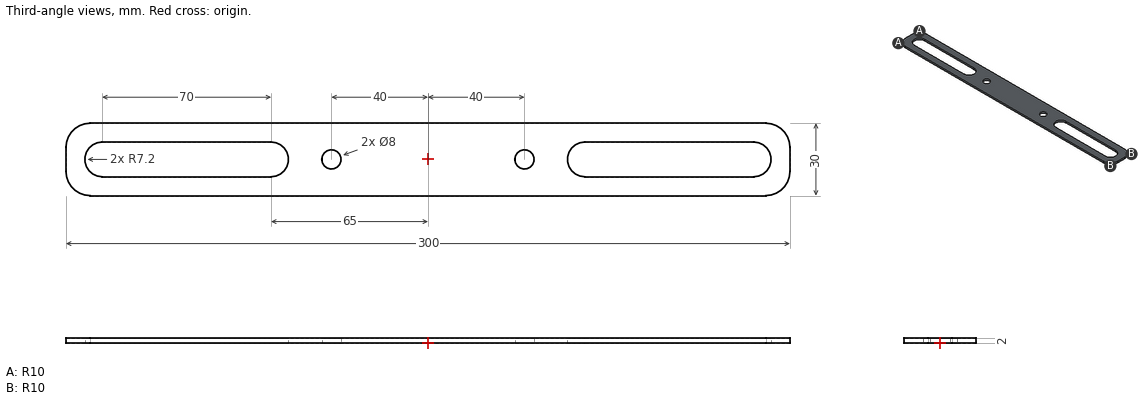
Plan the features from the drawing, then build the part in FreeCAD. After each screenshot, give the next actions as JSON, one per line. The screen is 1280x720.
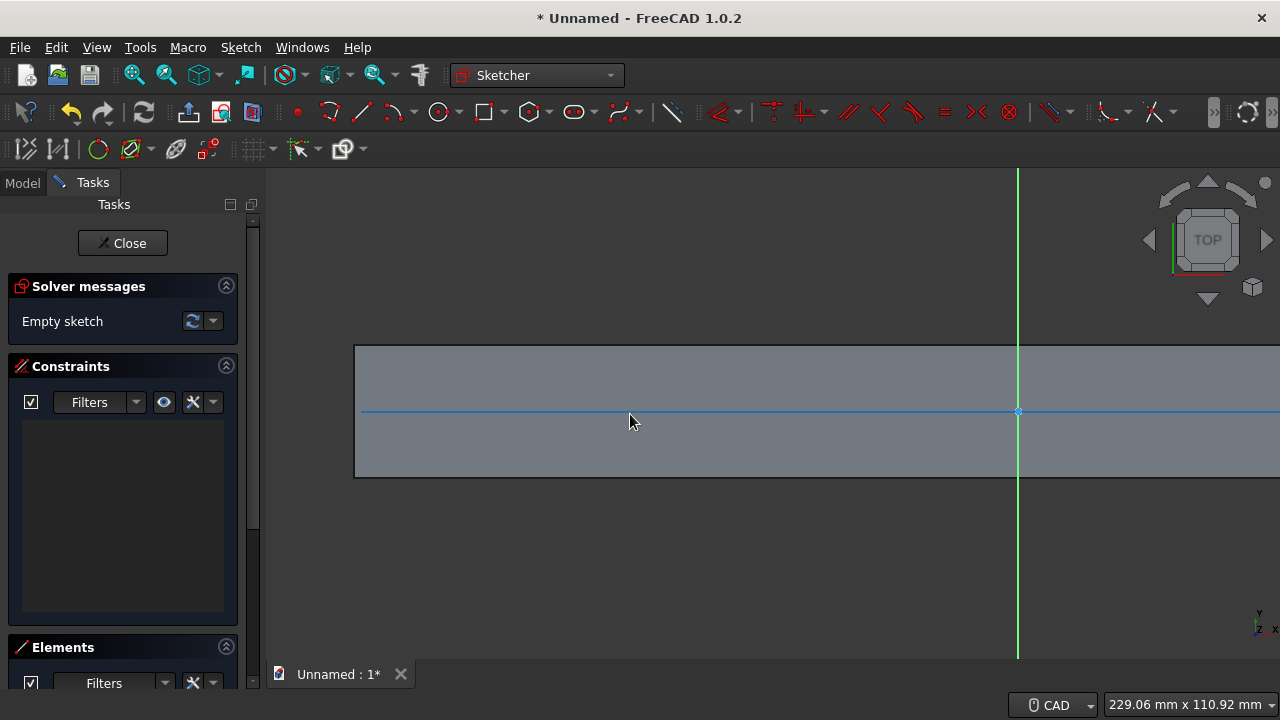
{"action": "key", "text": "g s"}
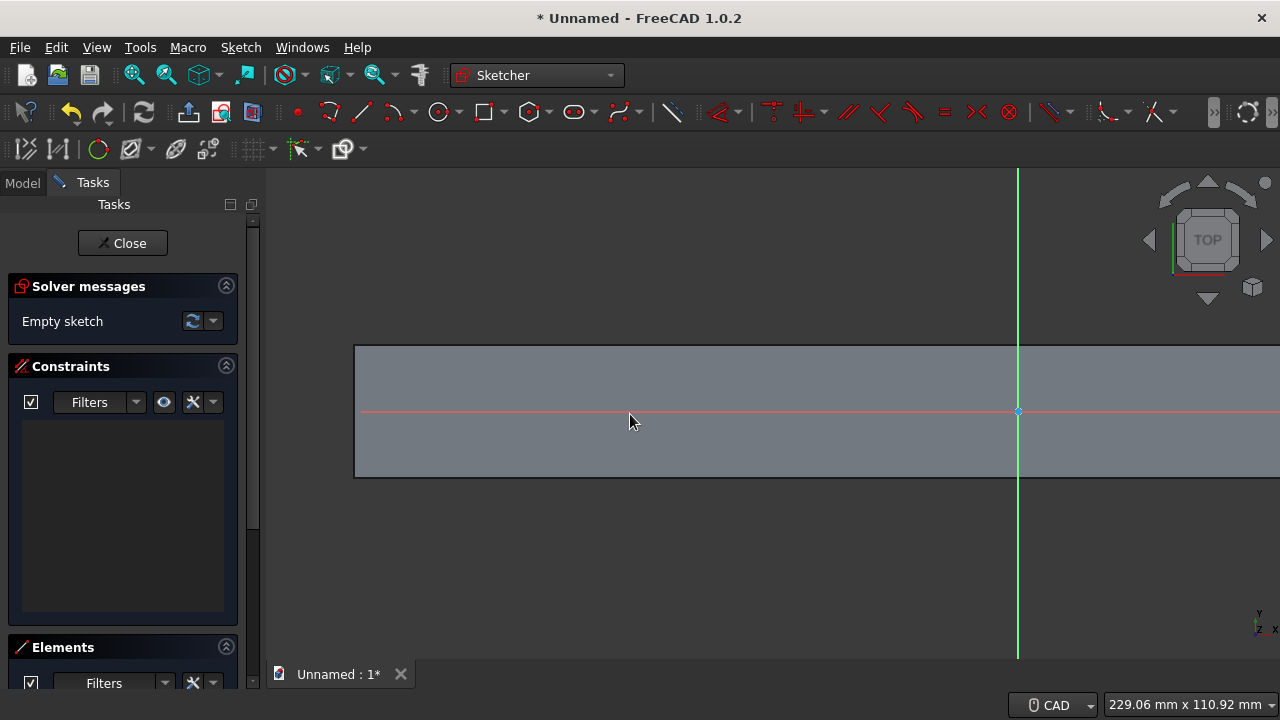
{"action": "left_click", "coordinate": [420, 412]}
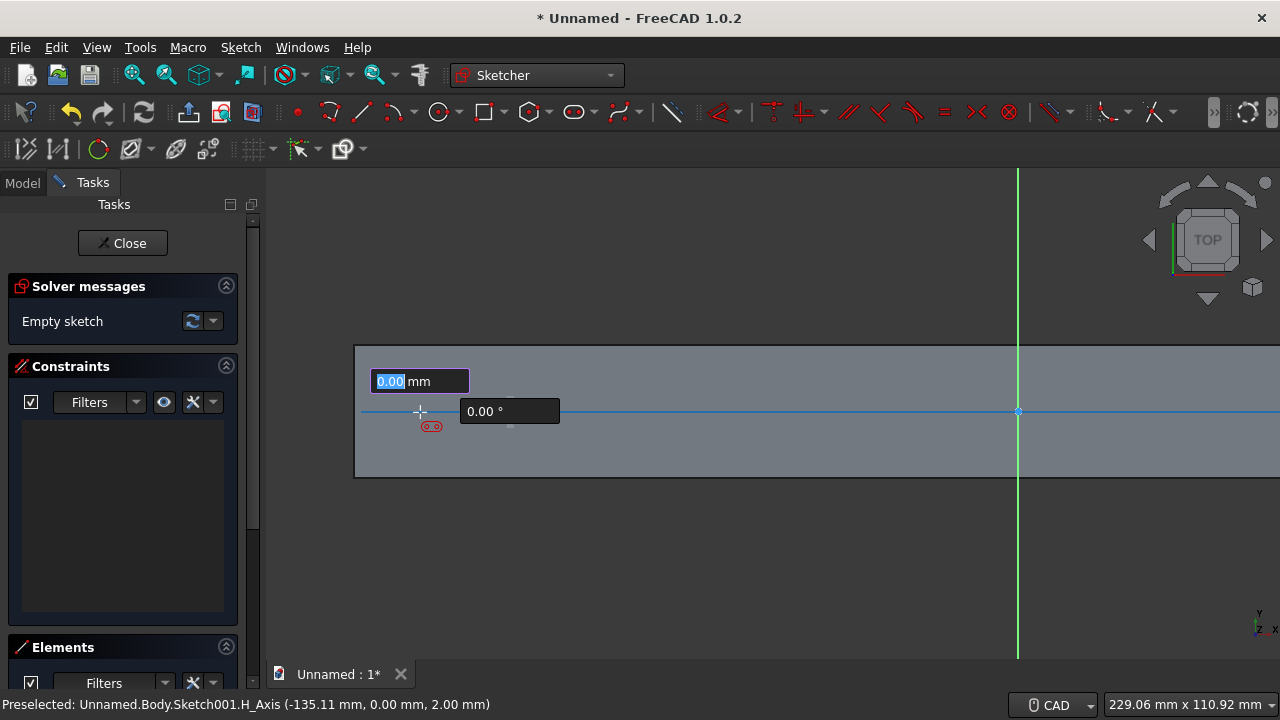
{"action": "left_click", "coordinate": [730, 403]}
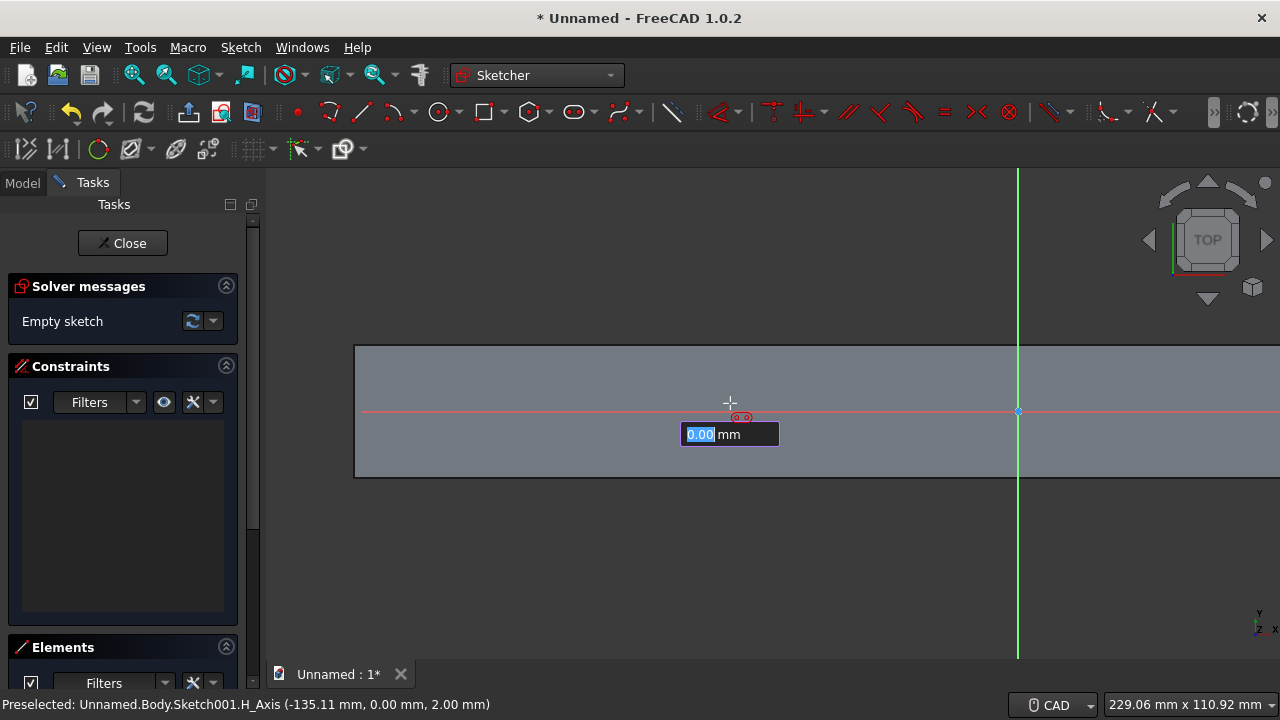
{"action": "left_click", "coordinate": [575, 380]}
{"action": "key", "text": "Escape"}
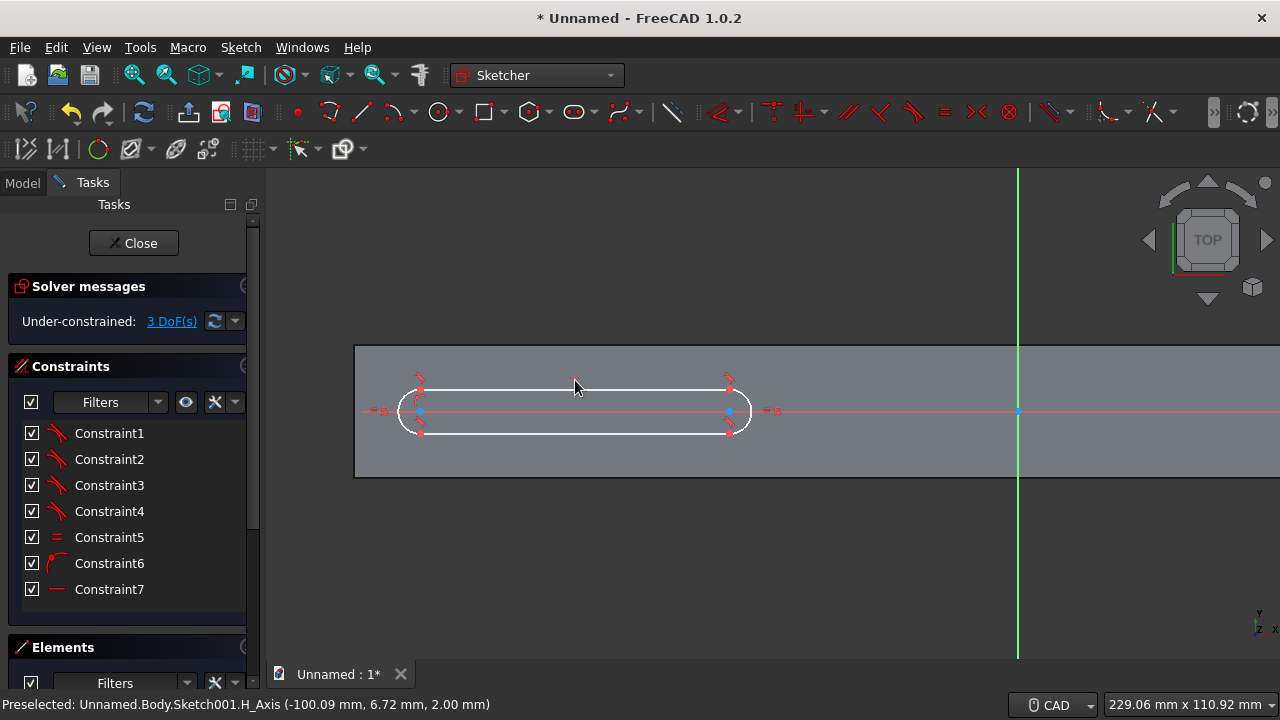
{"action": "scroll", "coordinate": [403, 399], "scroll_direction": "up", "scroll_amount": 2}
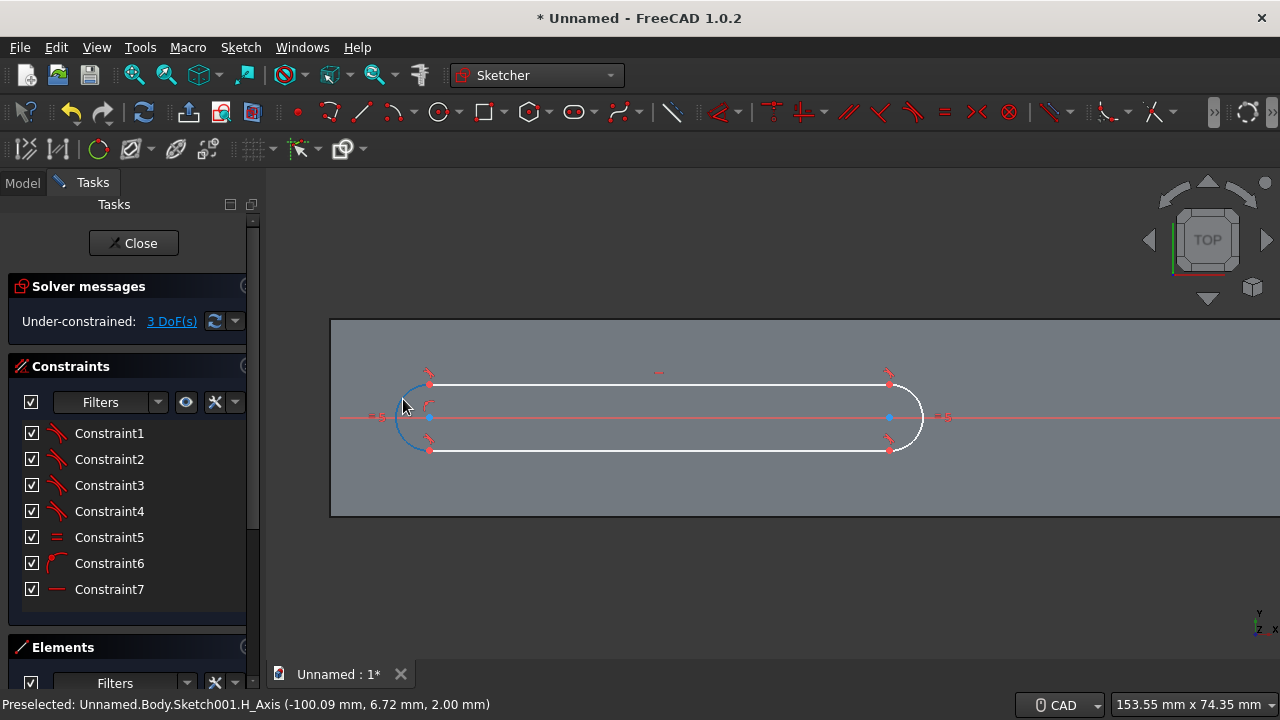
{"action": "left_click", "coordinate": [402, 398]}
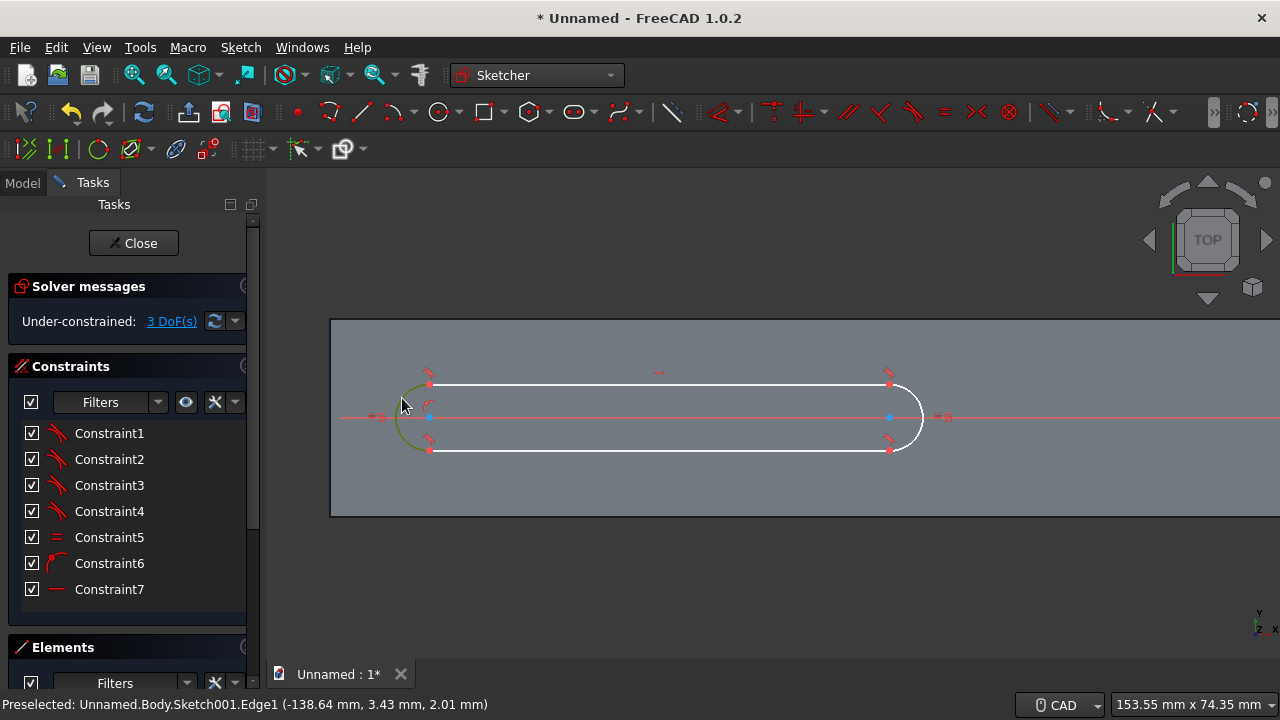
{"action": "key", "text": "k r"}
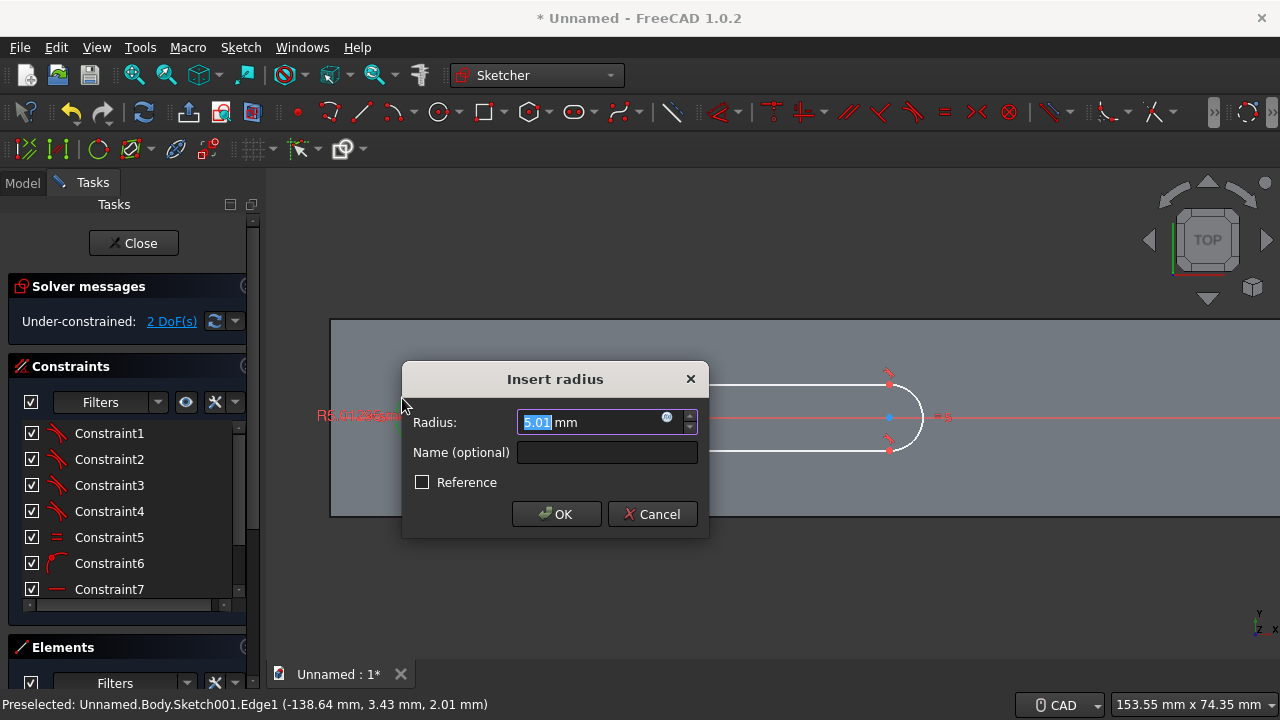
{"action": "type", "text": "7.2"}
{"action": "key", "text": "Return"}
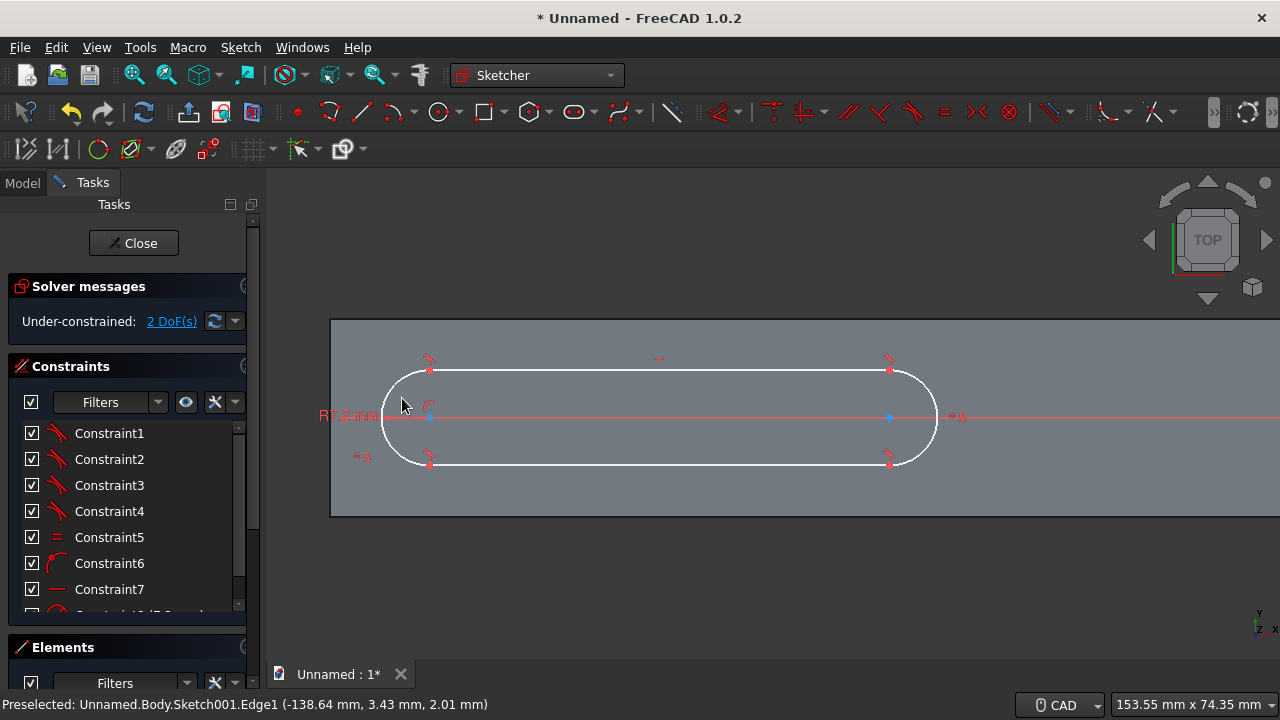
{"action": "left_click", "coordinate": [567, 370]}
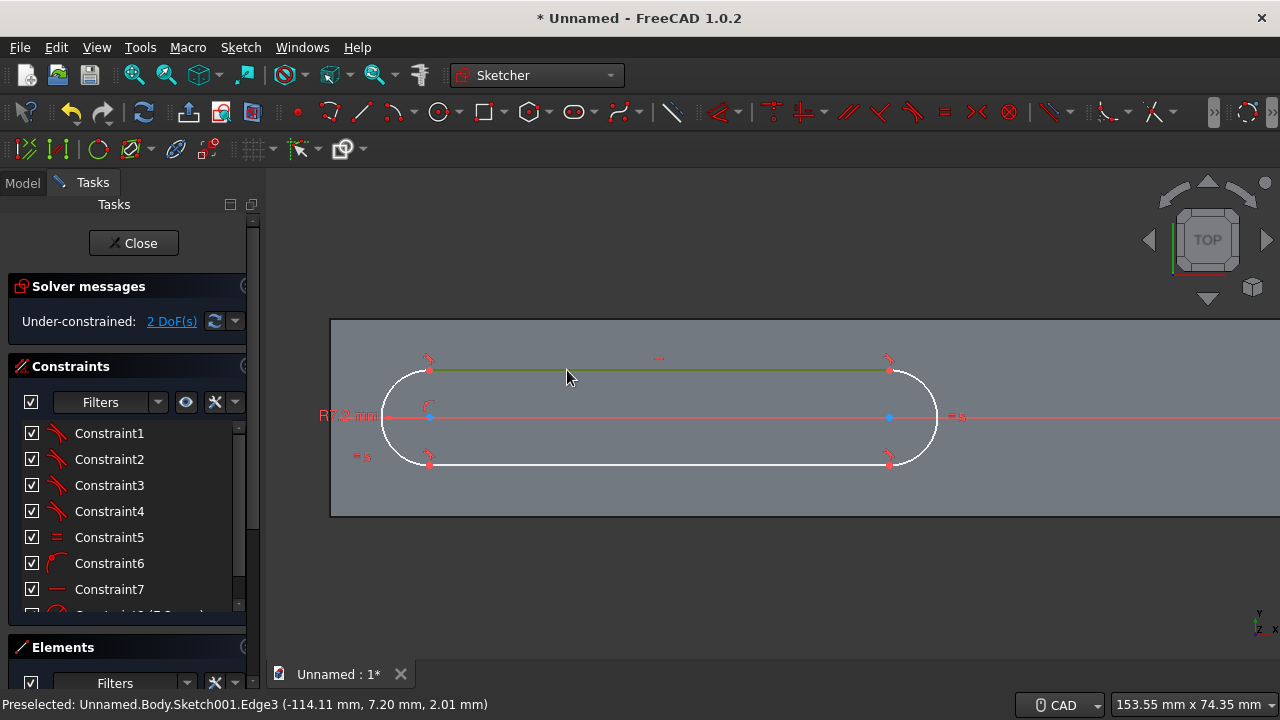
{"action": "key", "text": "l"}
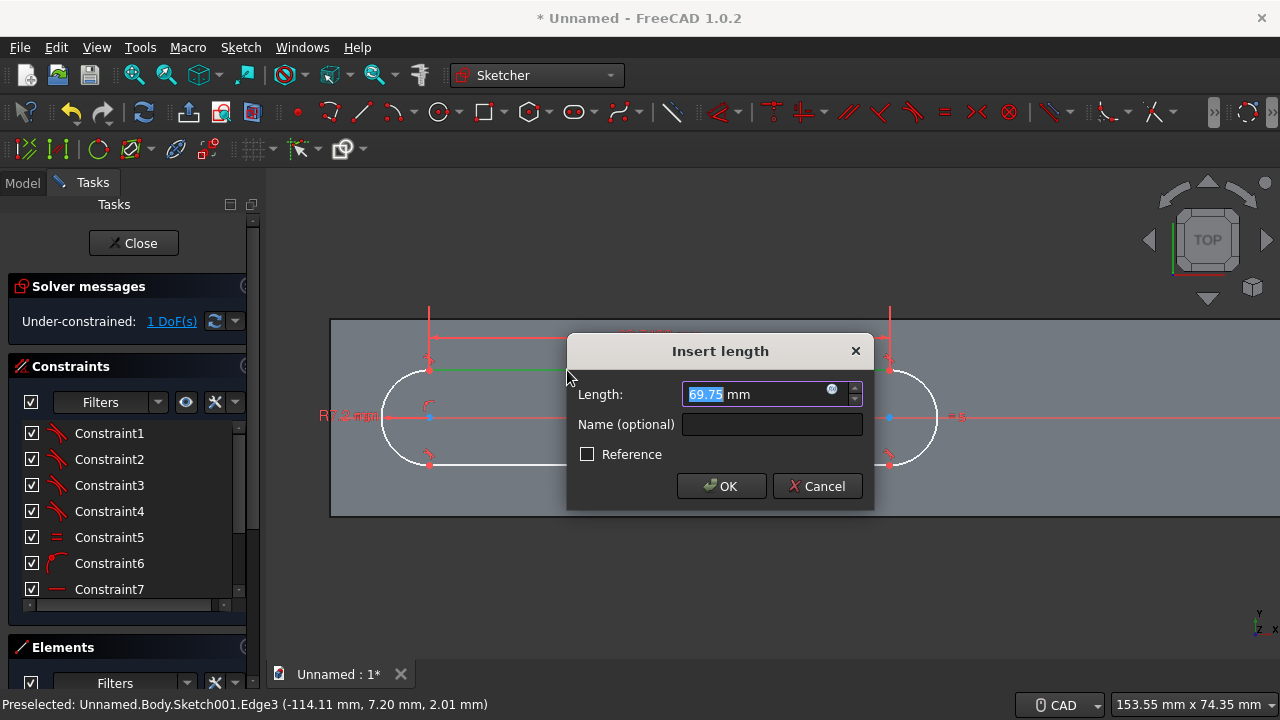
{"action": "type", "text": "70"}
{"action": "key", "text": "Return"}